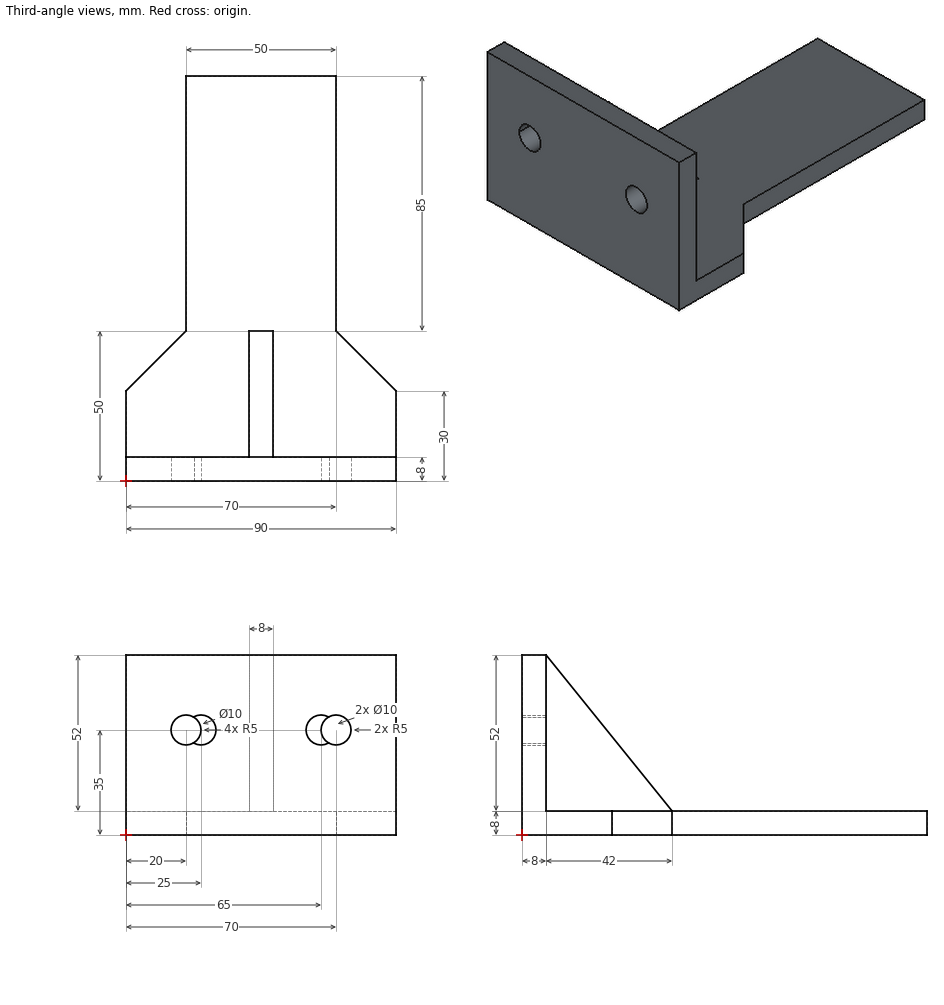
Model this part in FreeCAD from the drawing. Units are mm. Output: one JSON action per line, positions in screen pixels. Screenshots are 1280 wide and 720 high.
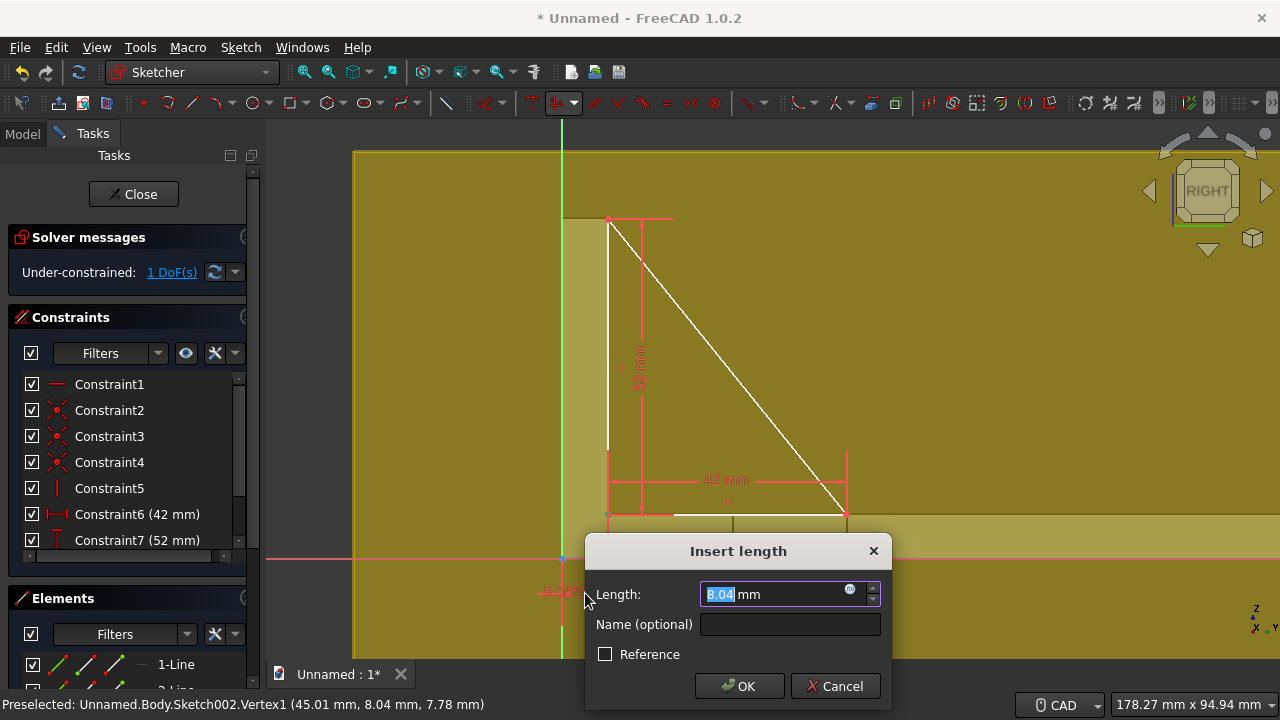
{"action": "type", "text": "8"}
{"action": "key", "text": "Return"}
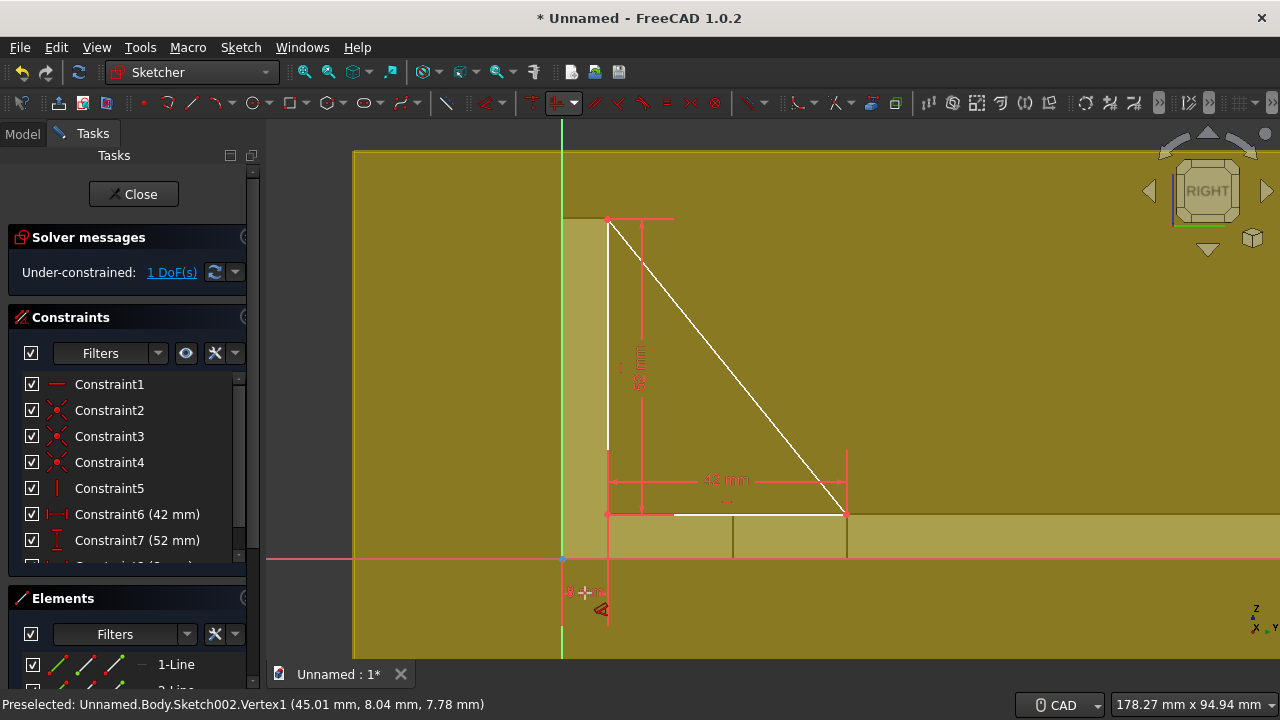
{"action": "left_click", "coordinate": [608, 515]}
{"action": "left_click", "coordinate": [528, 537]}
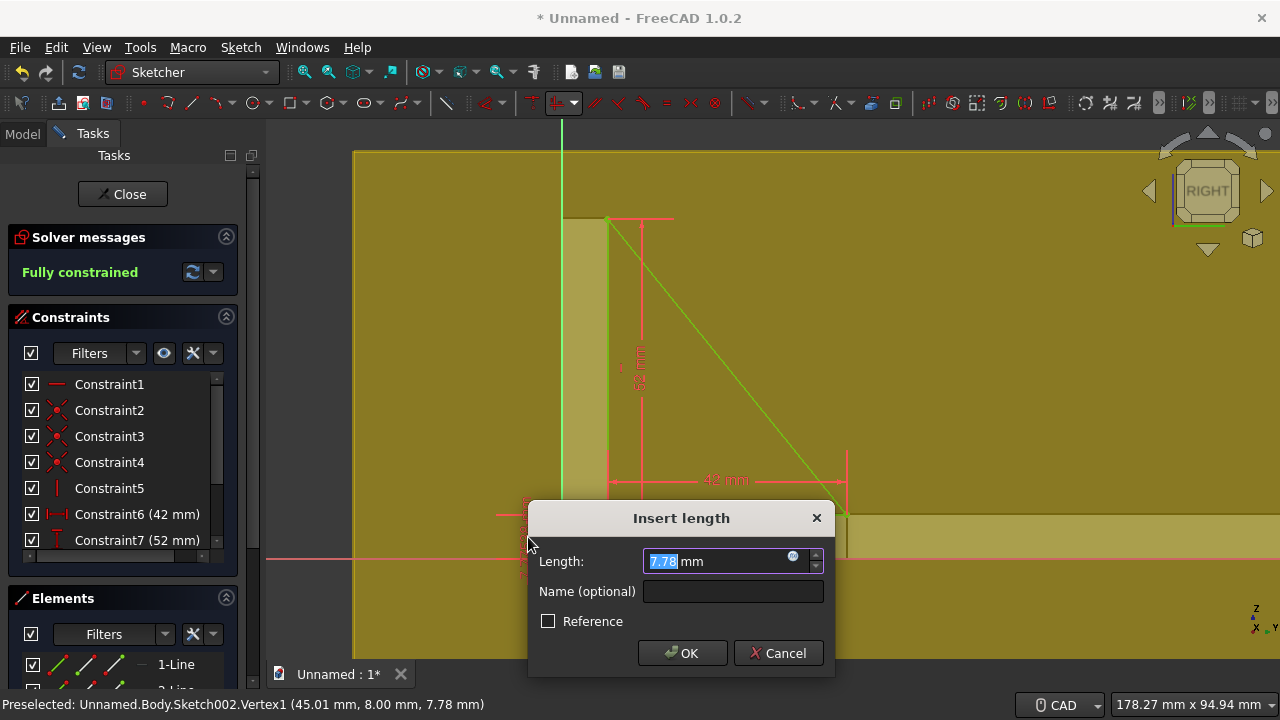
{"action": "type", "text": "8"}
{"action": "key", "text": "Return"}
{"action": "key", "text": "Escape"}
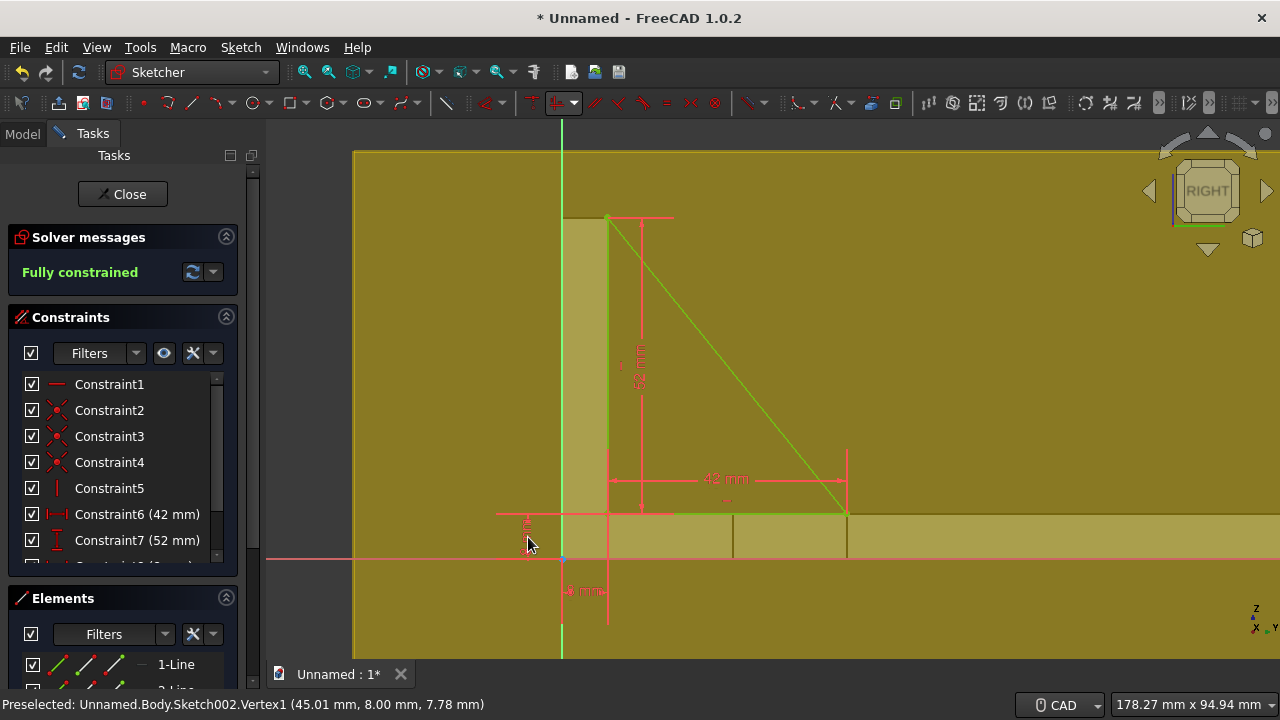
{"action": "left_click", "coordinate": [123, 194]}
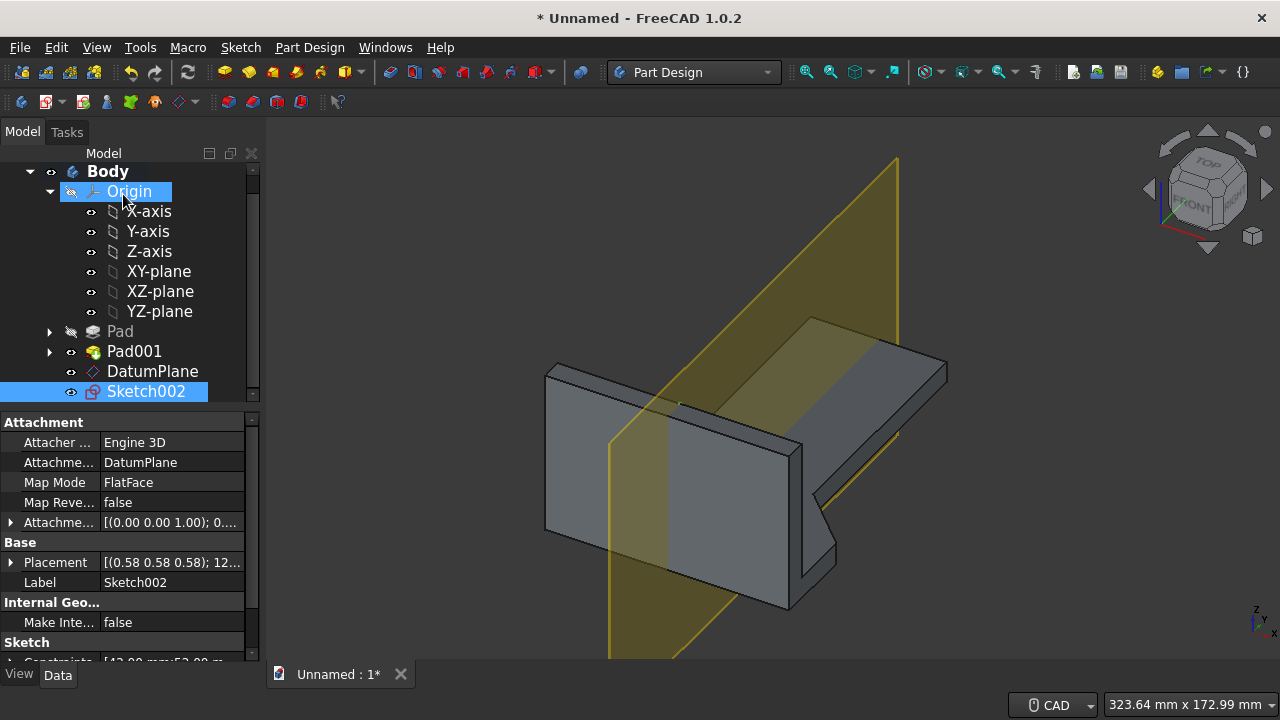
{"action": "left_click", "coordinate": [226, 72]}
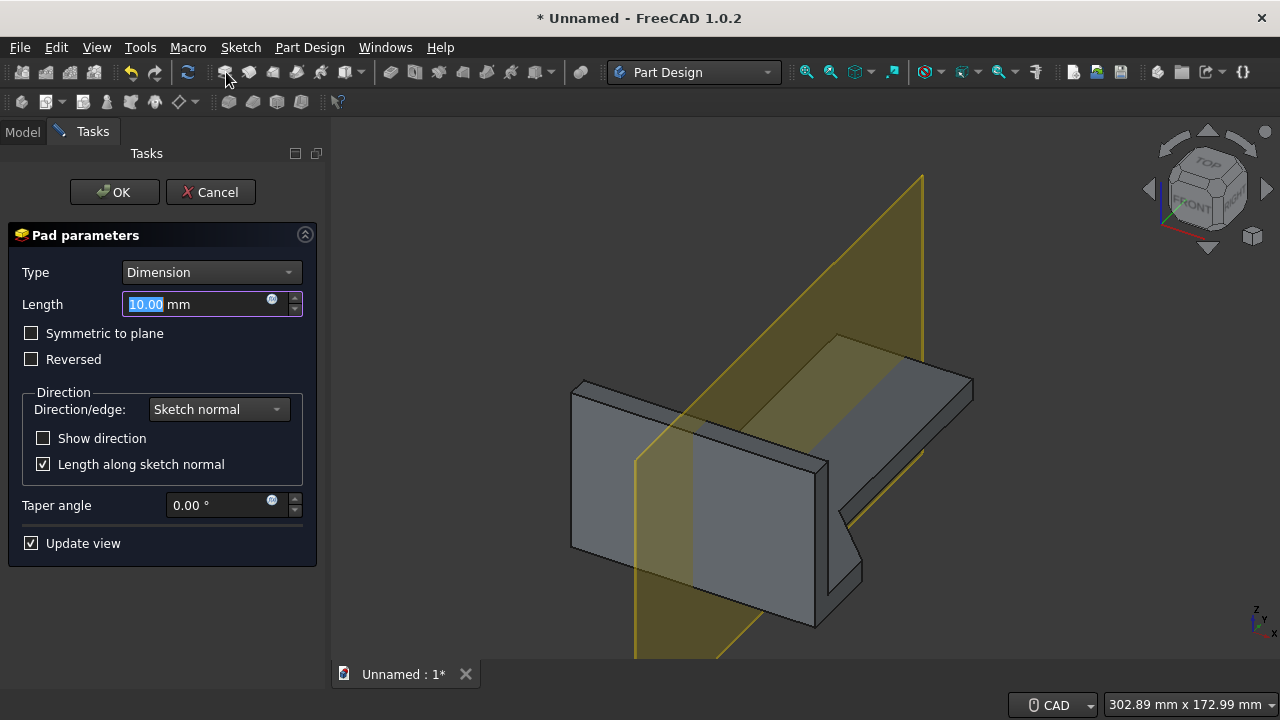
{"action": "type", "text": "8"}
{"action": "key", "text": "Tab"}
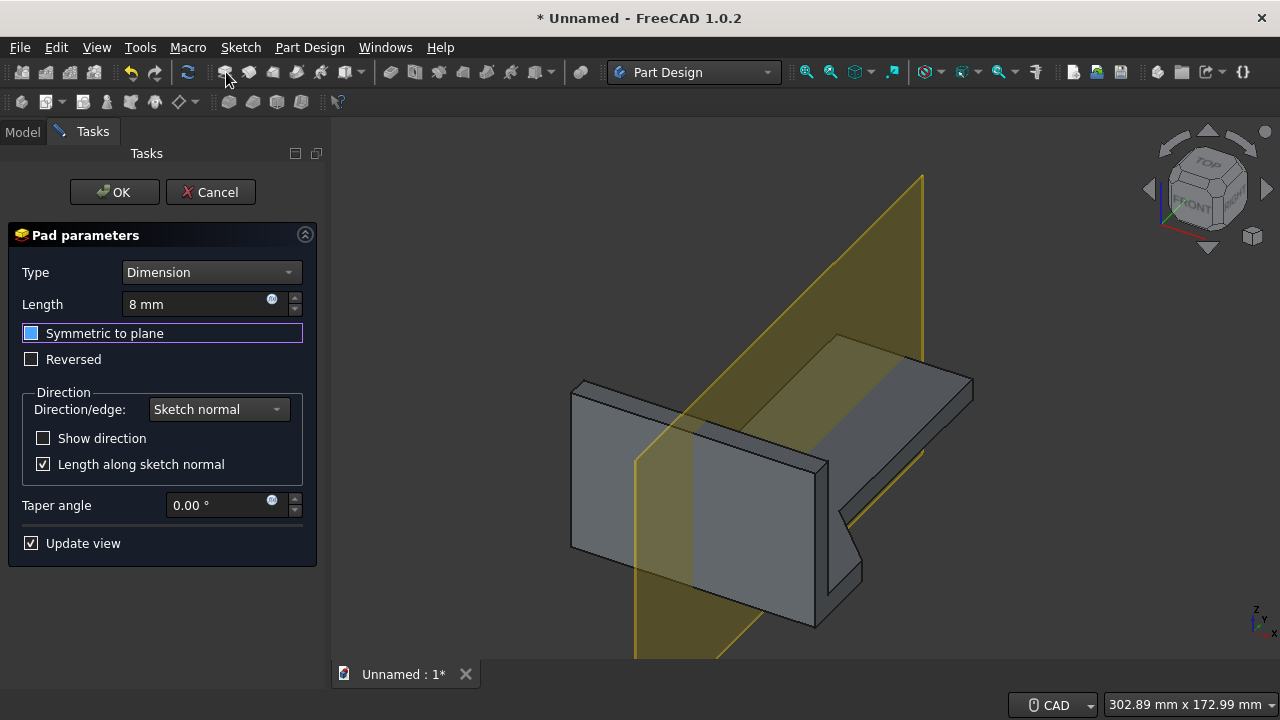
{"action": "left_click", "coordinate": [30, 333]}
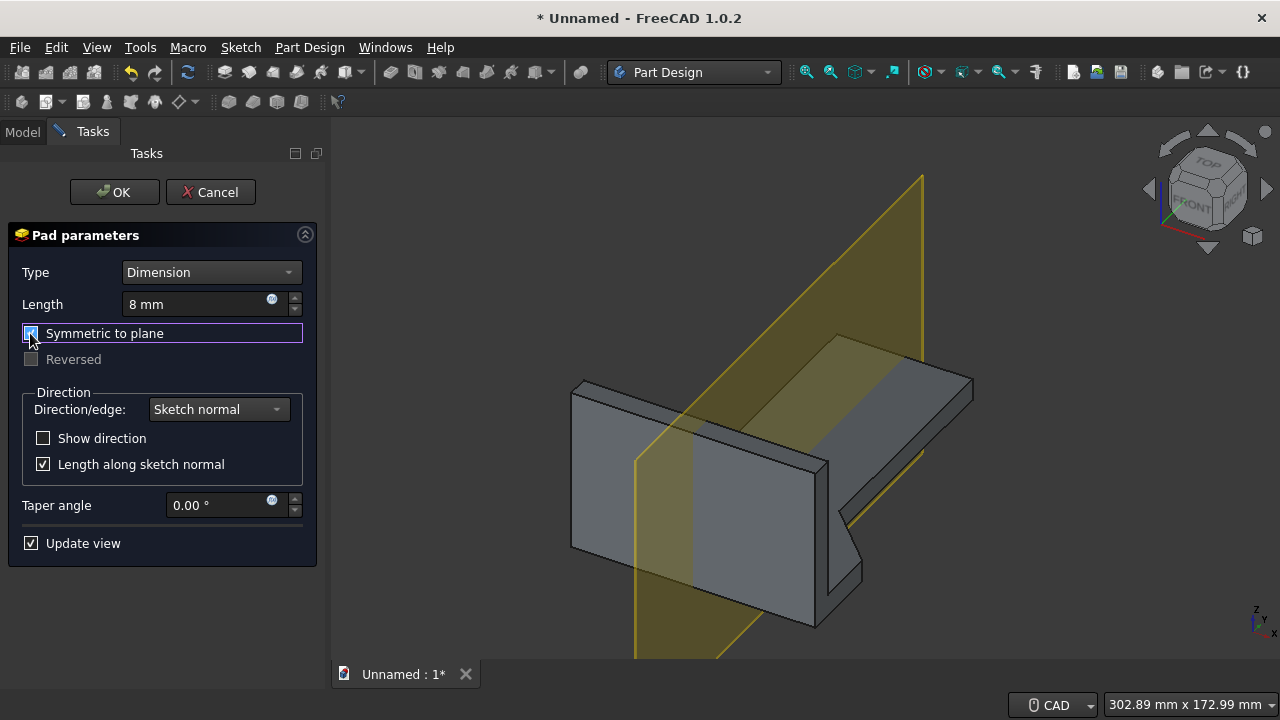
{"action": "left_click", "coordinate": [115, 192]}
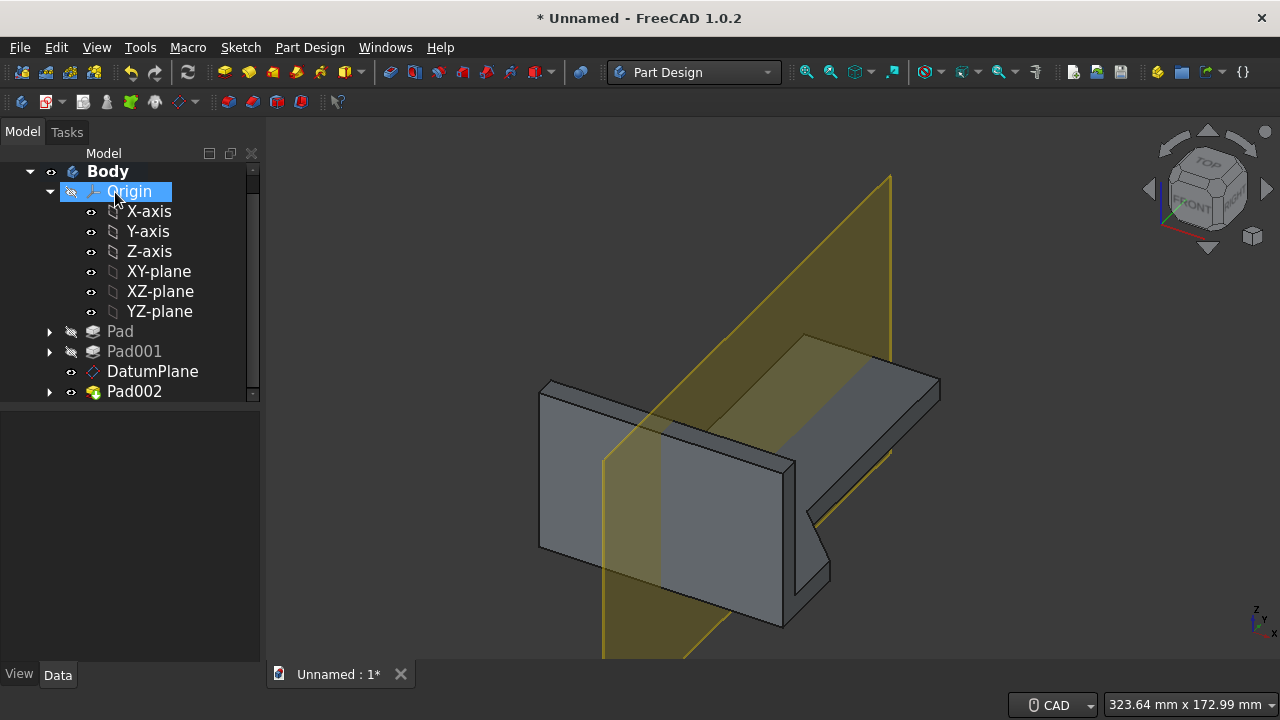
{"action": "left_click", "coordinate": [116, 372]}
{"action": "key", "text": "space"}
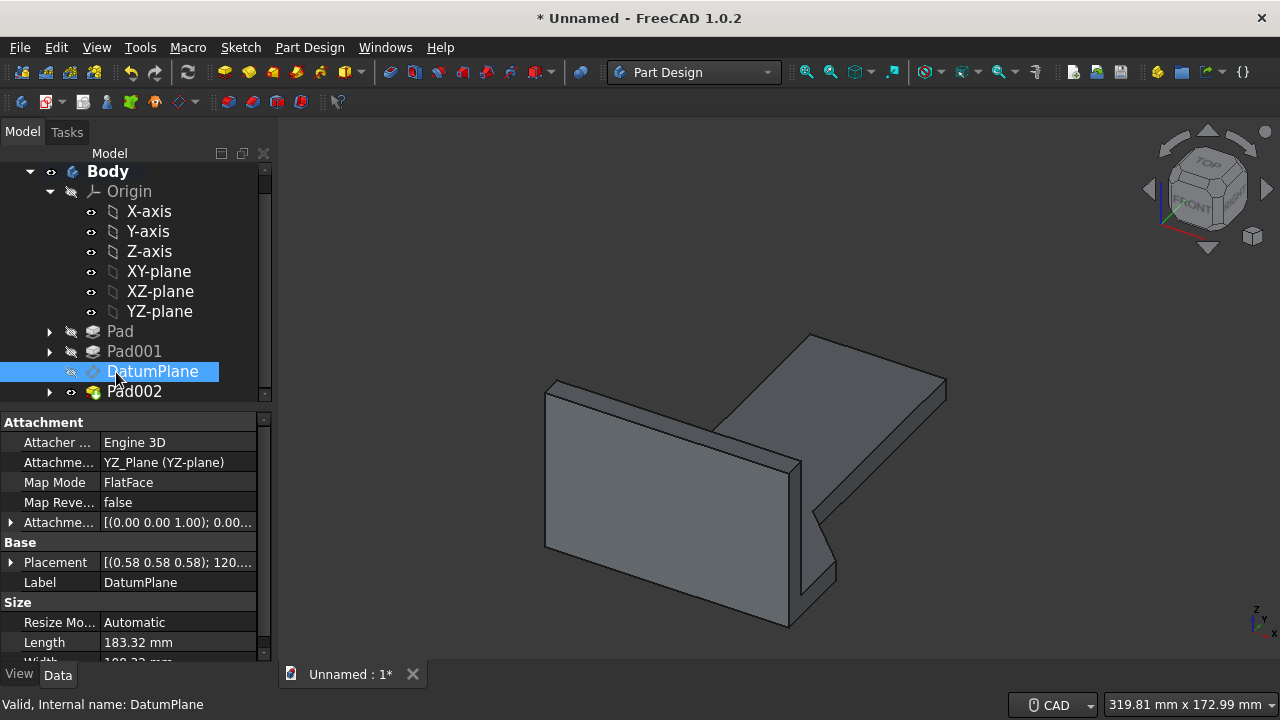
{"action": "key", "text": "4"}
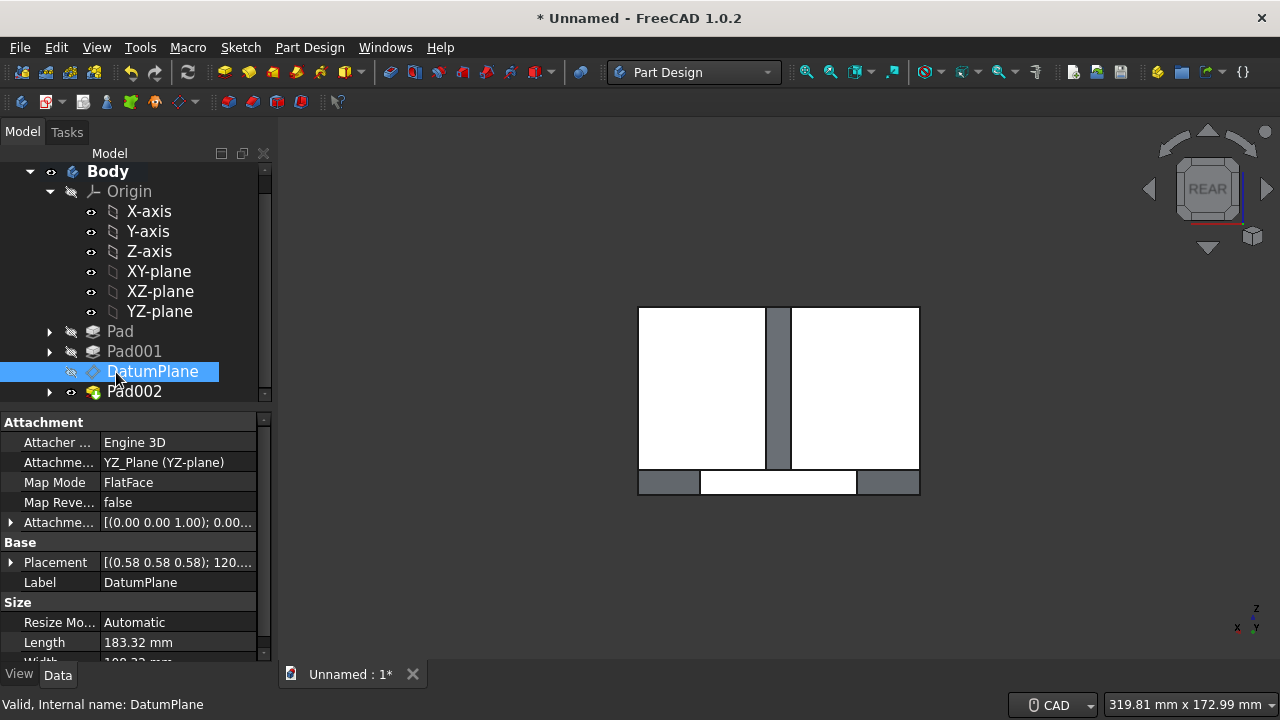
{"action": "left_click", "coordinate": [808, 72]}